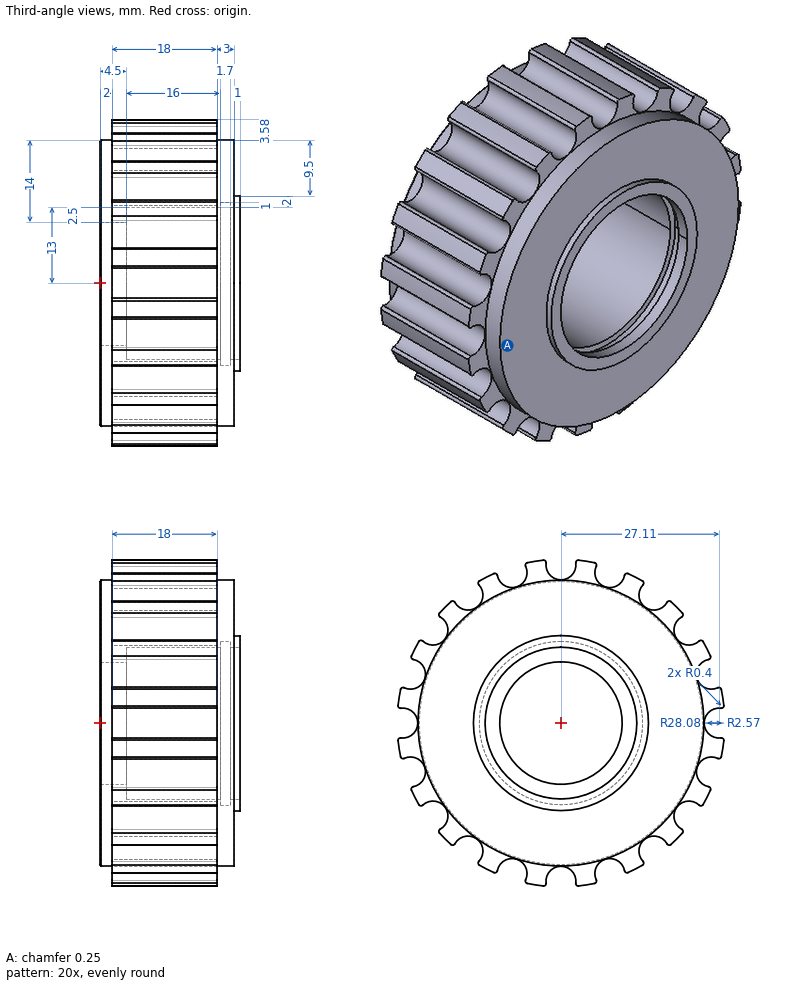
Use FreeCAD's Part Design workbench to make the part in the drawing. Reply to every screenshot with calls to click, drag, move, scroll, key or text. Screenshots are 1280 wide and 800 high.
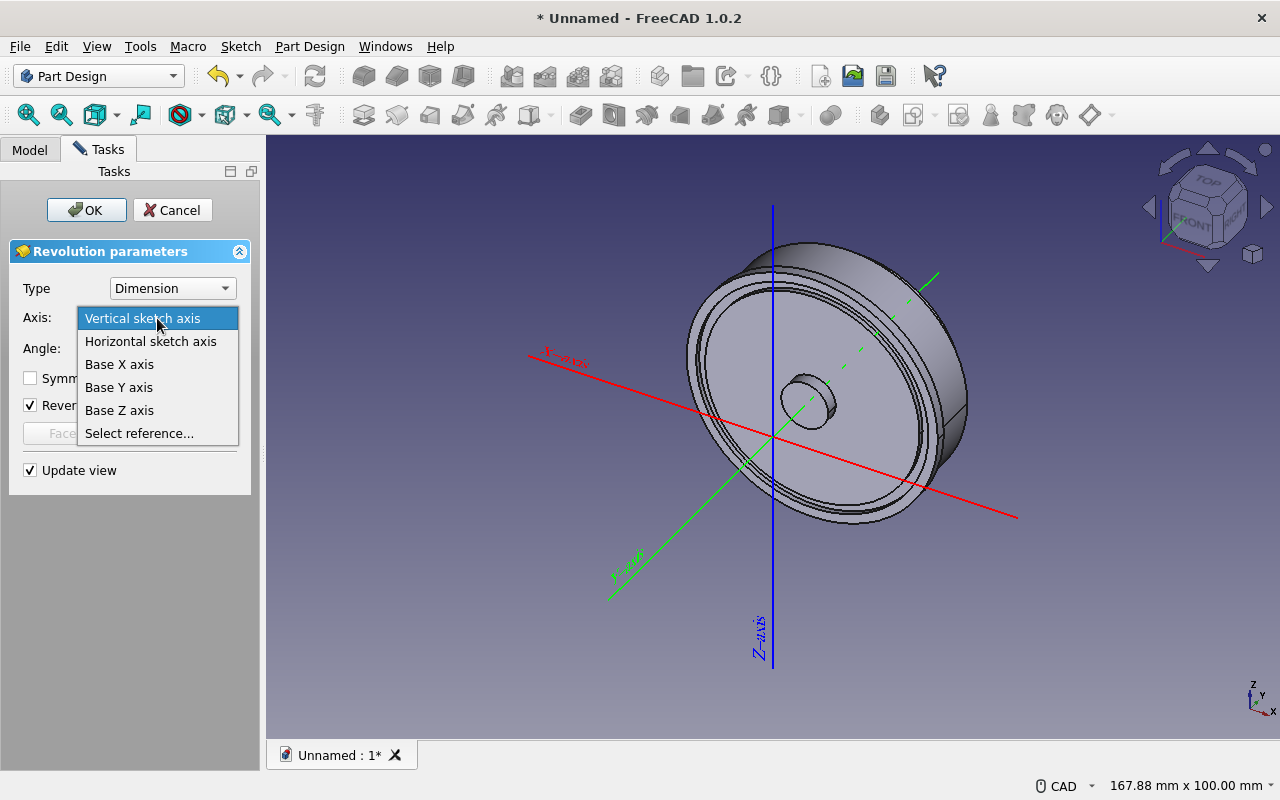
click(156, 342)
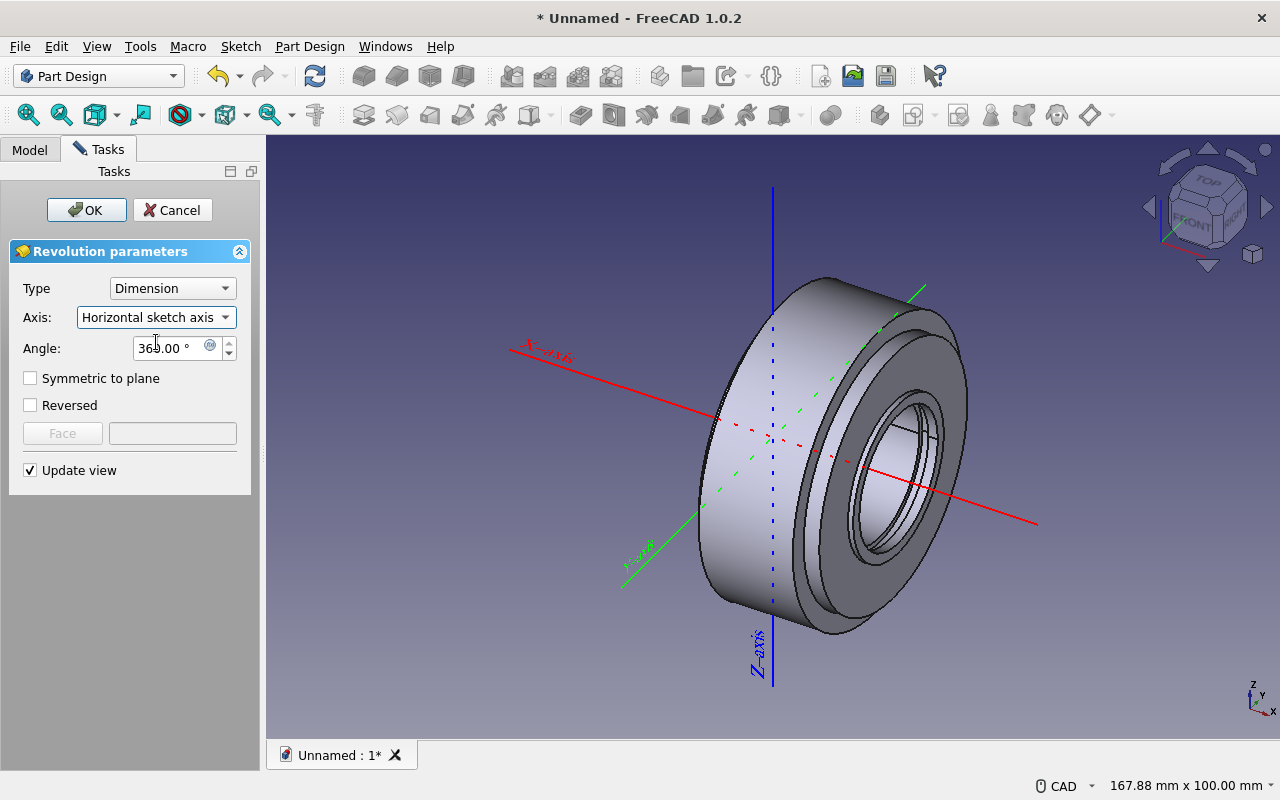
click(87, 210)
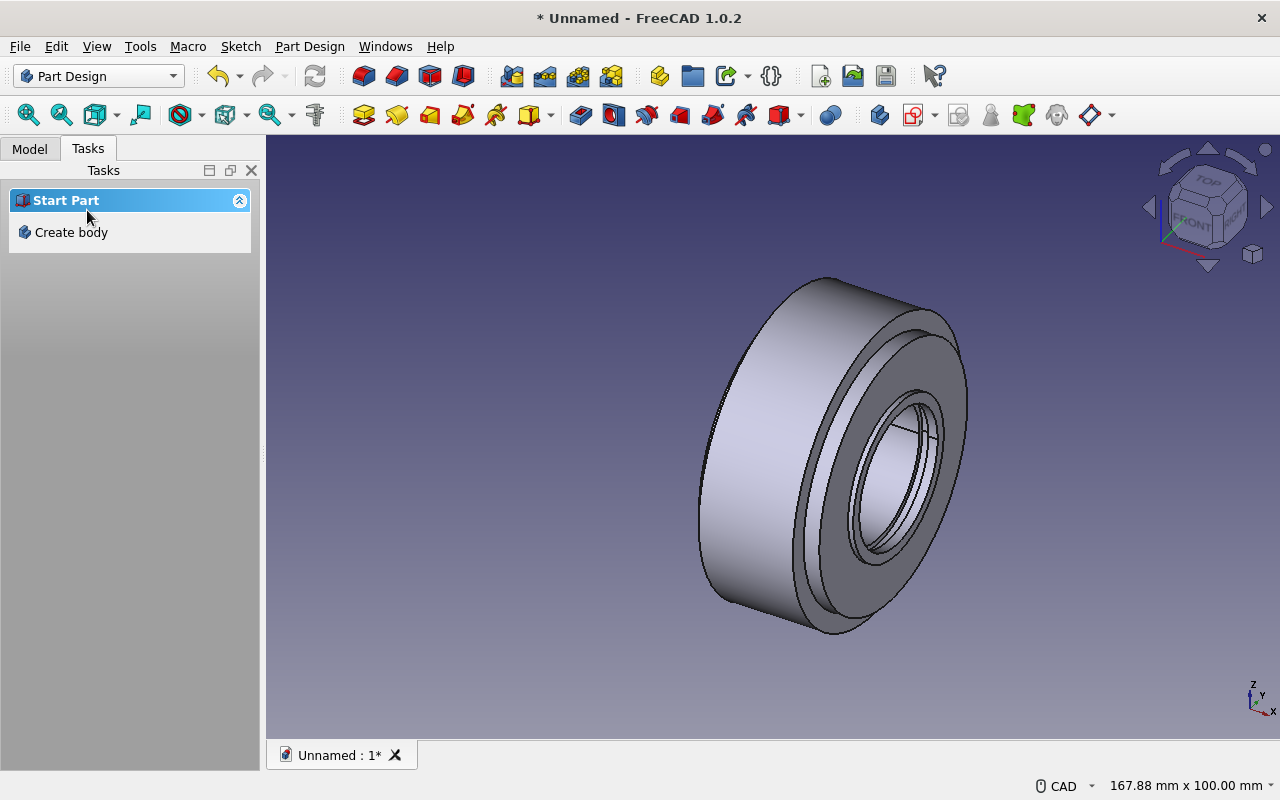
key(0)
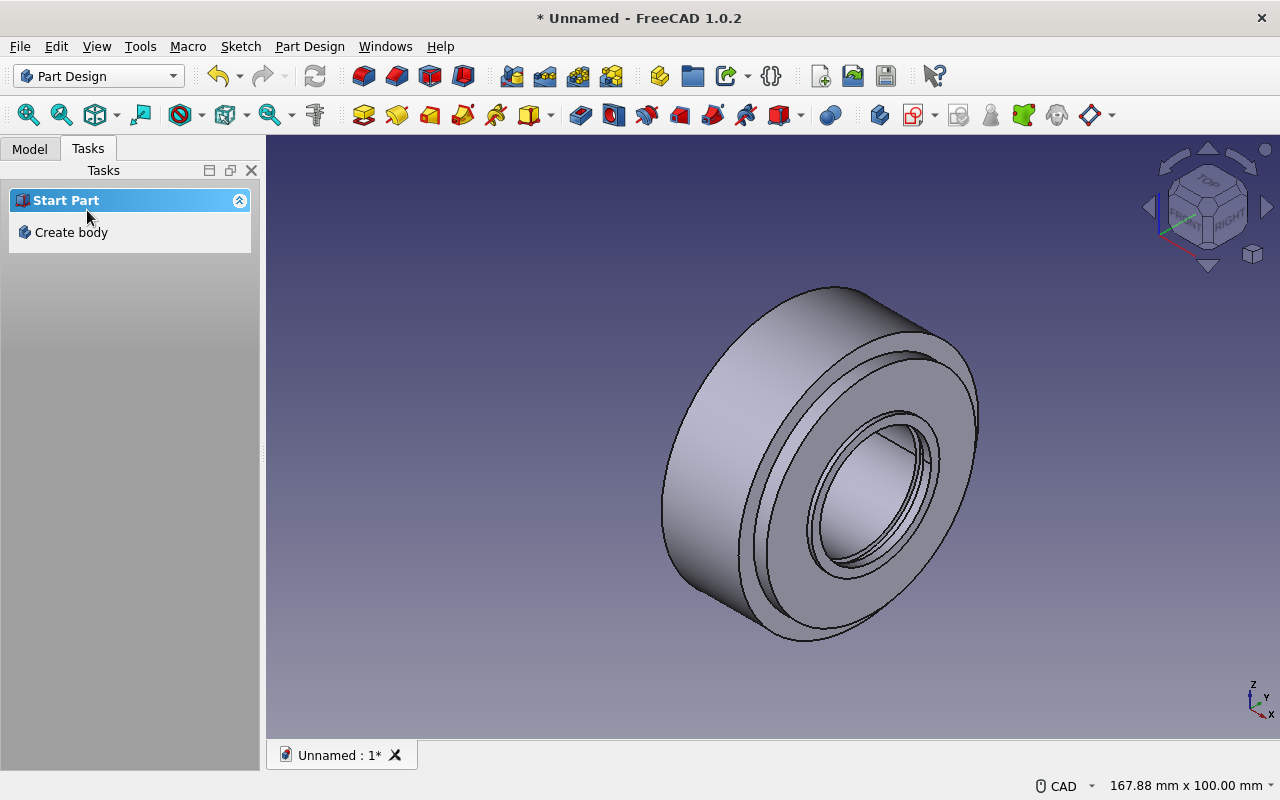
key(2)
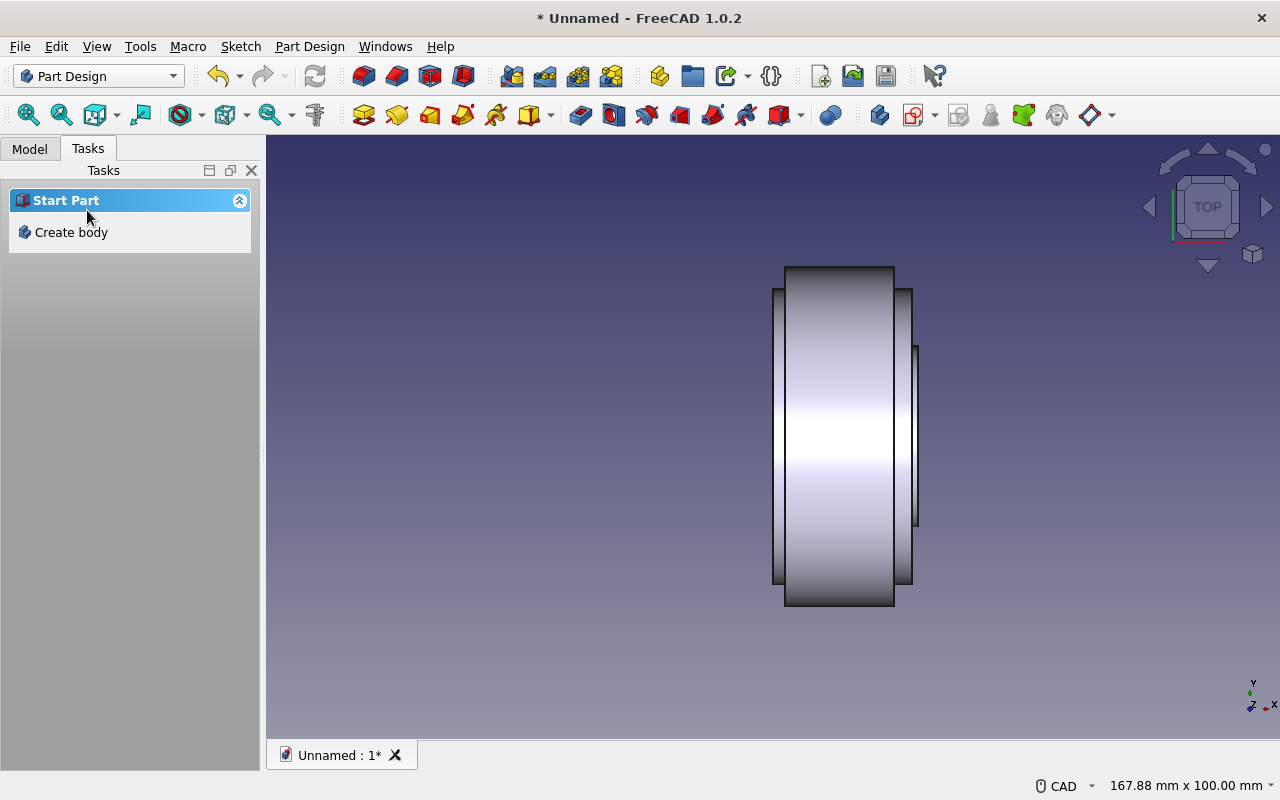
click(773, 556)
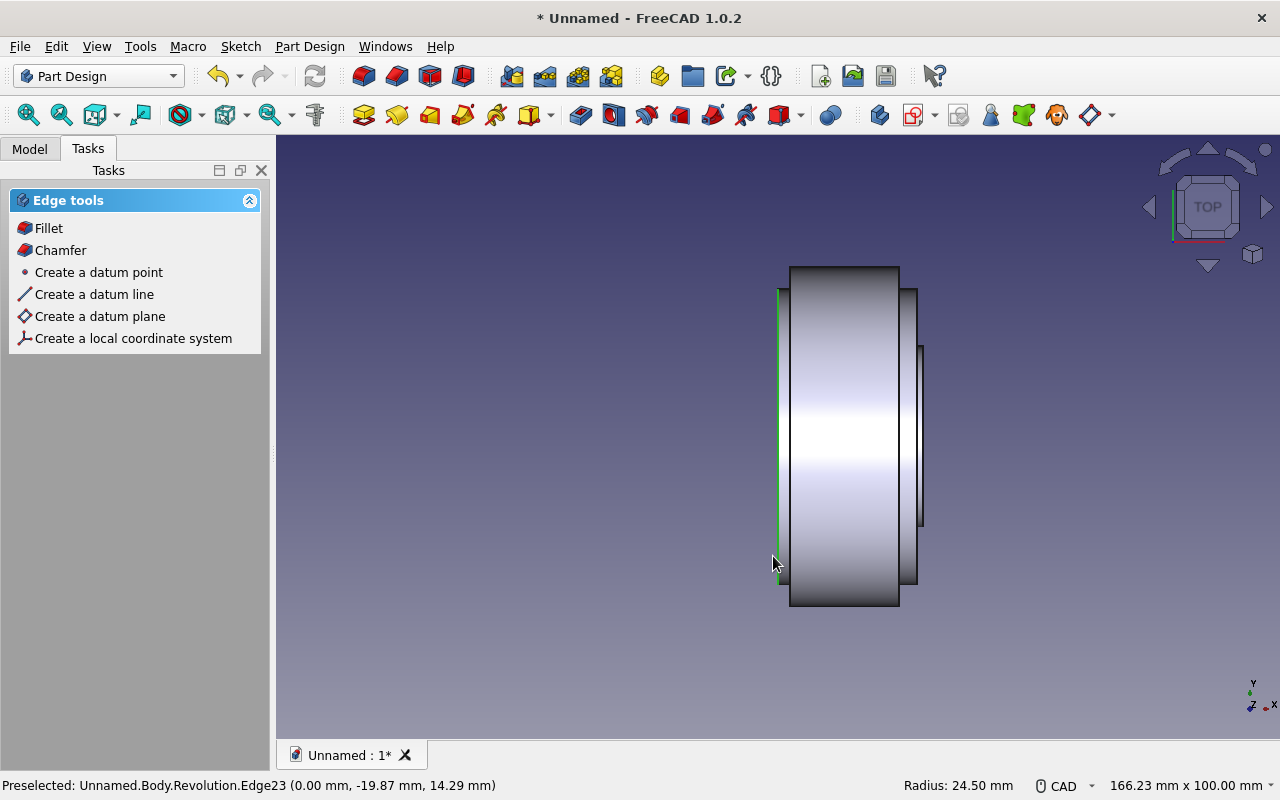
click(397, 76)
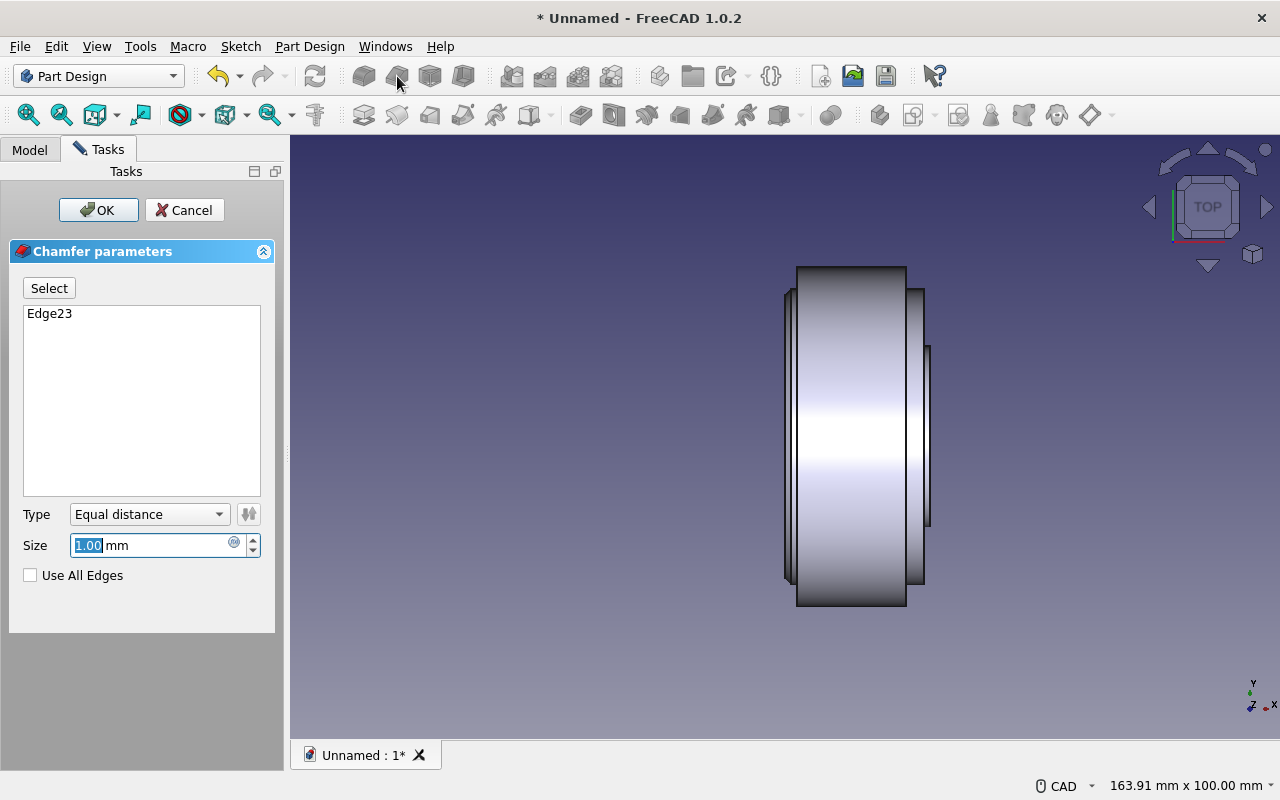
text(0.25)
key(Tab)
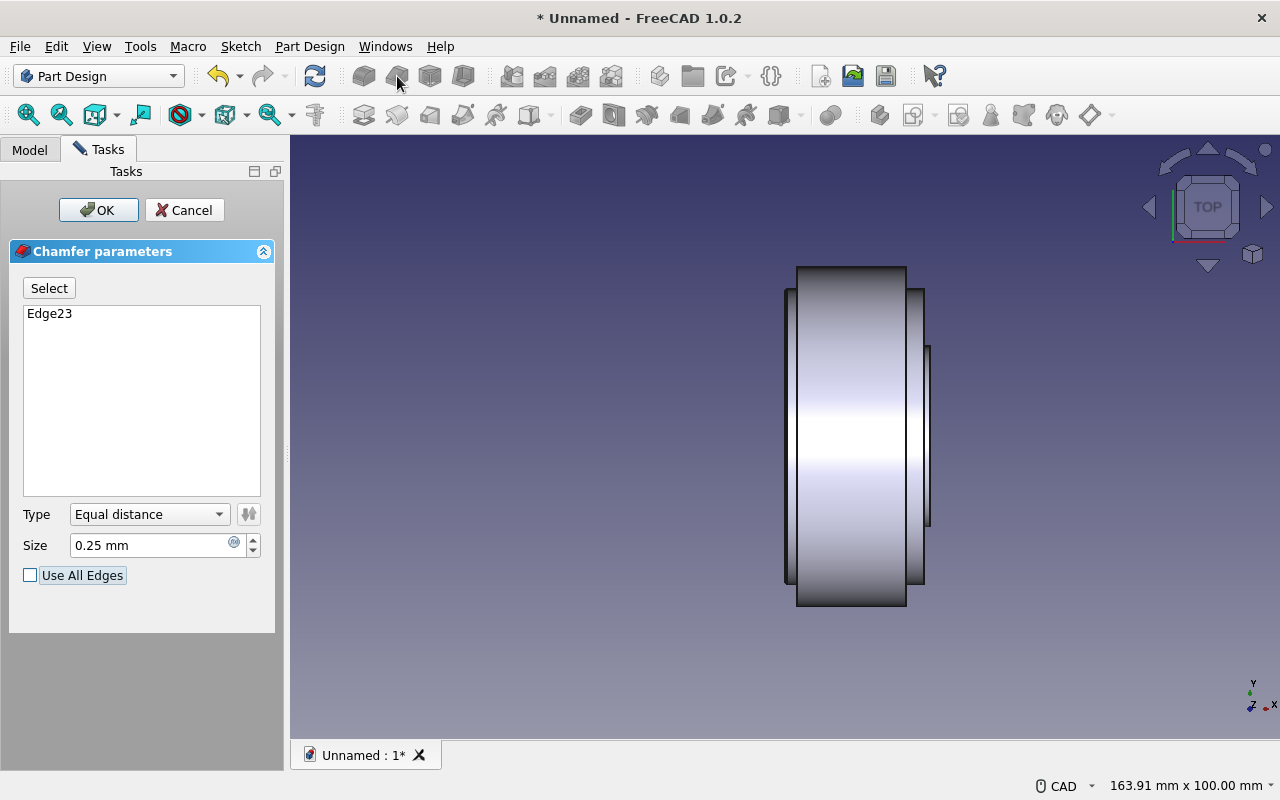
click(99, 210)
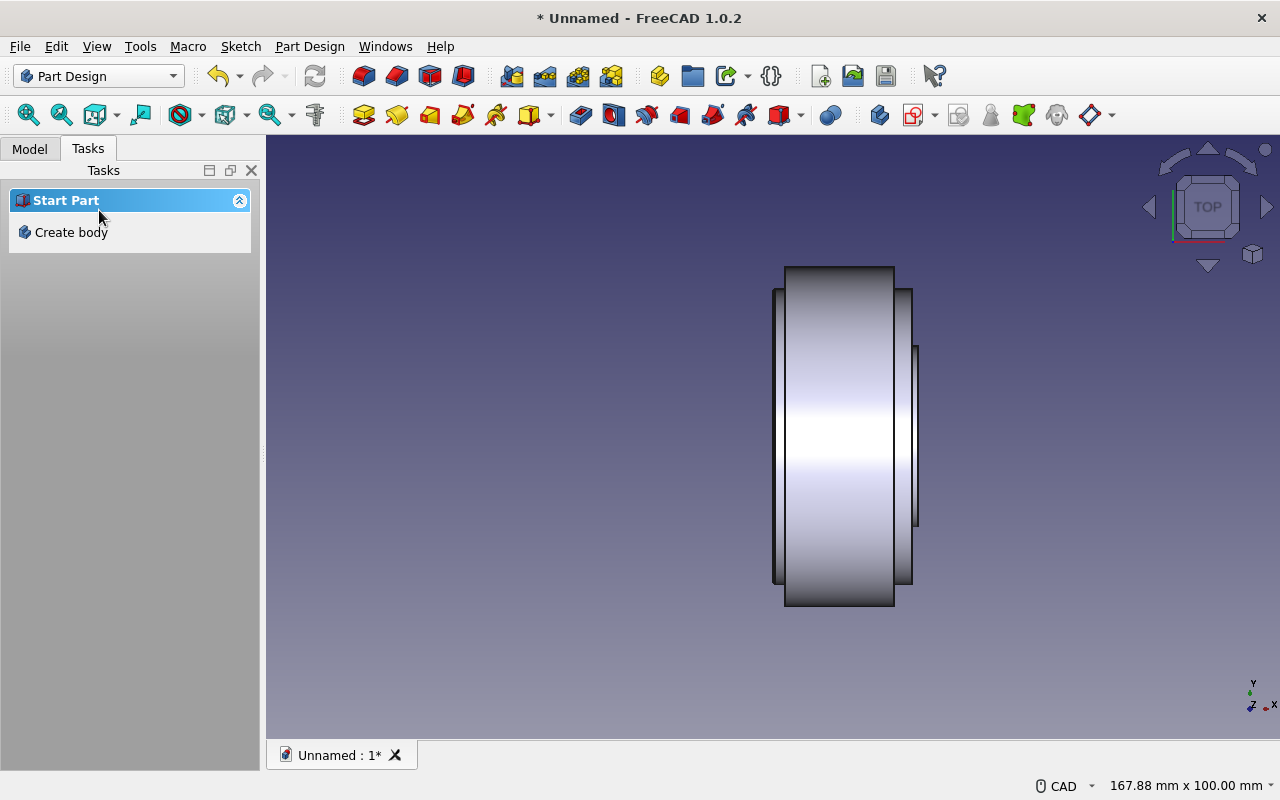
key(6)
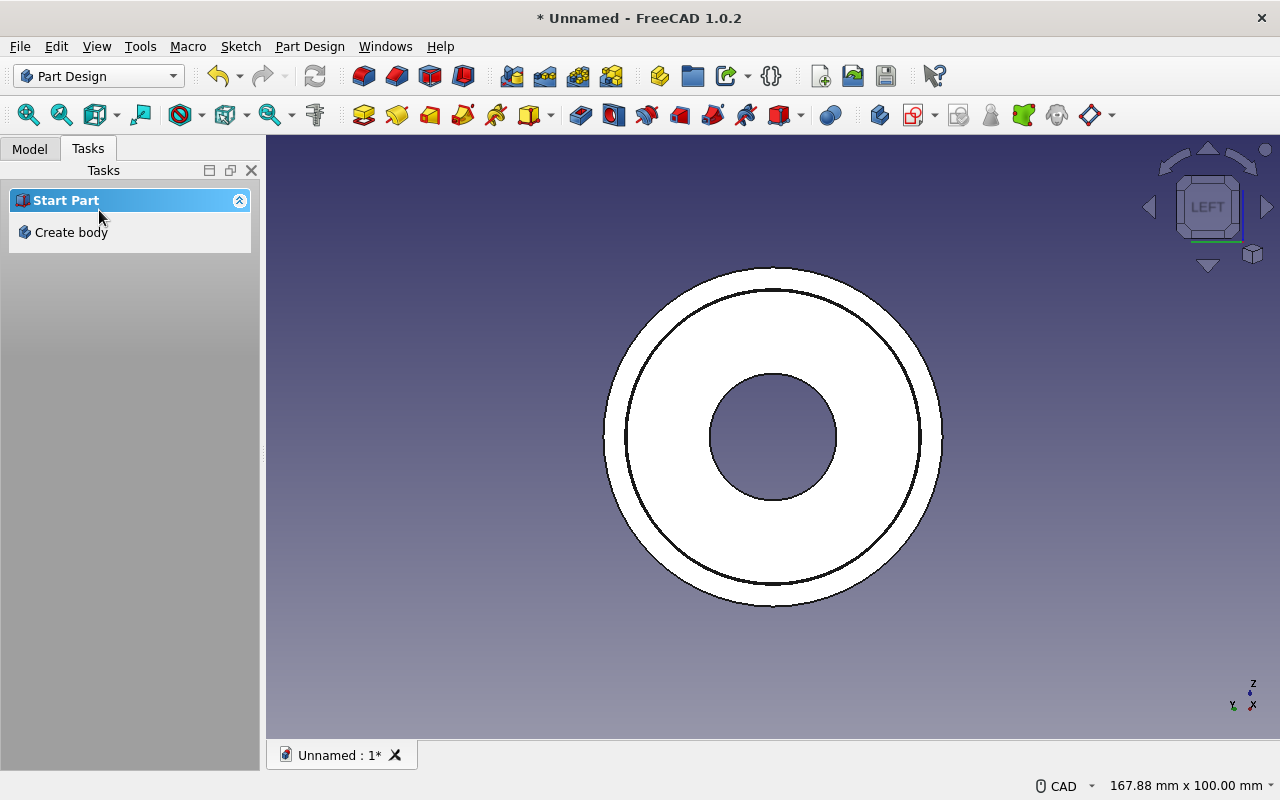
scroll(821, 581, up, 5)